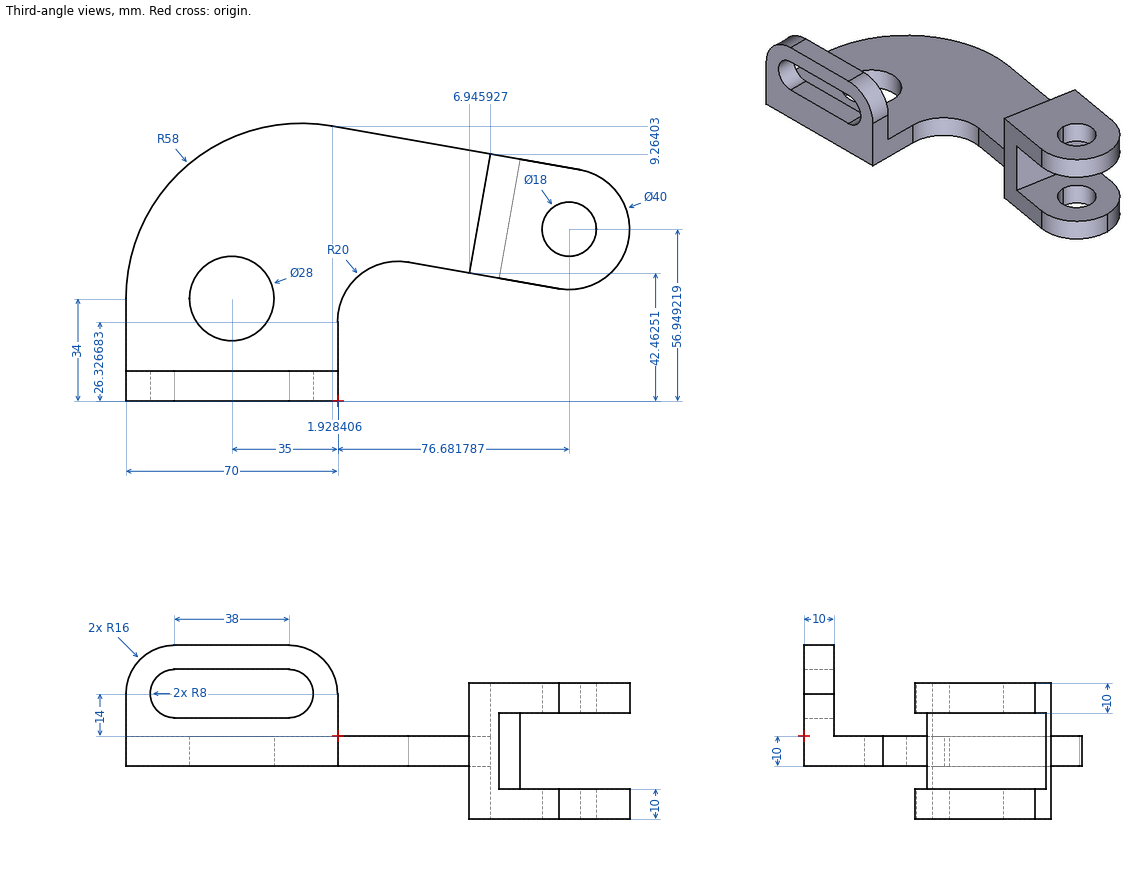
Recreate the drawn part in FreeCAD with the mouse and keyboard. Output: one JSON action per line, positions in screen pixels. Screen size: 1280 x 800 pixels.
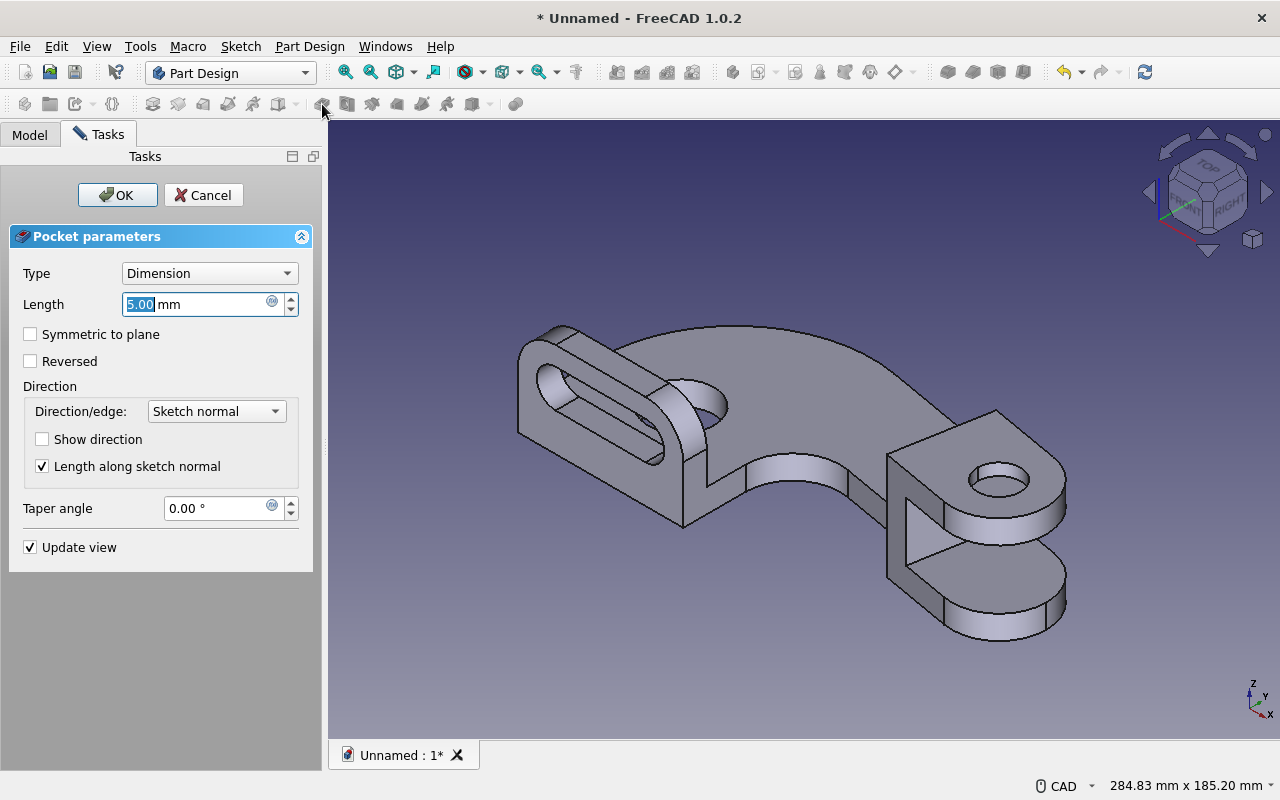
{"action": "left_click", "coordinate": [210, 274]}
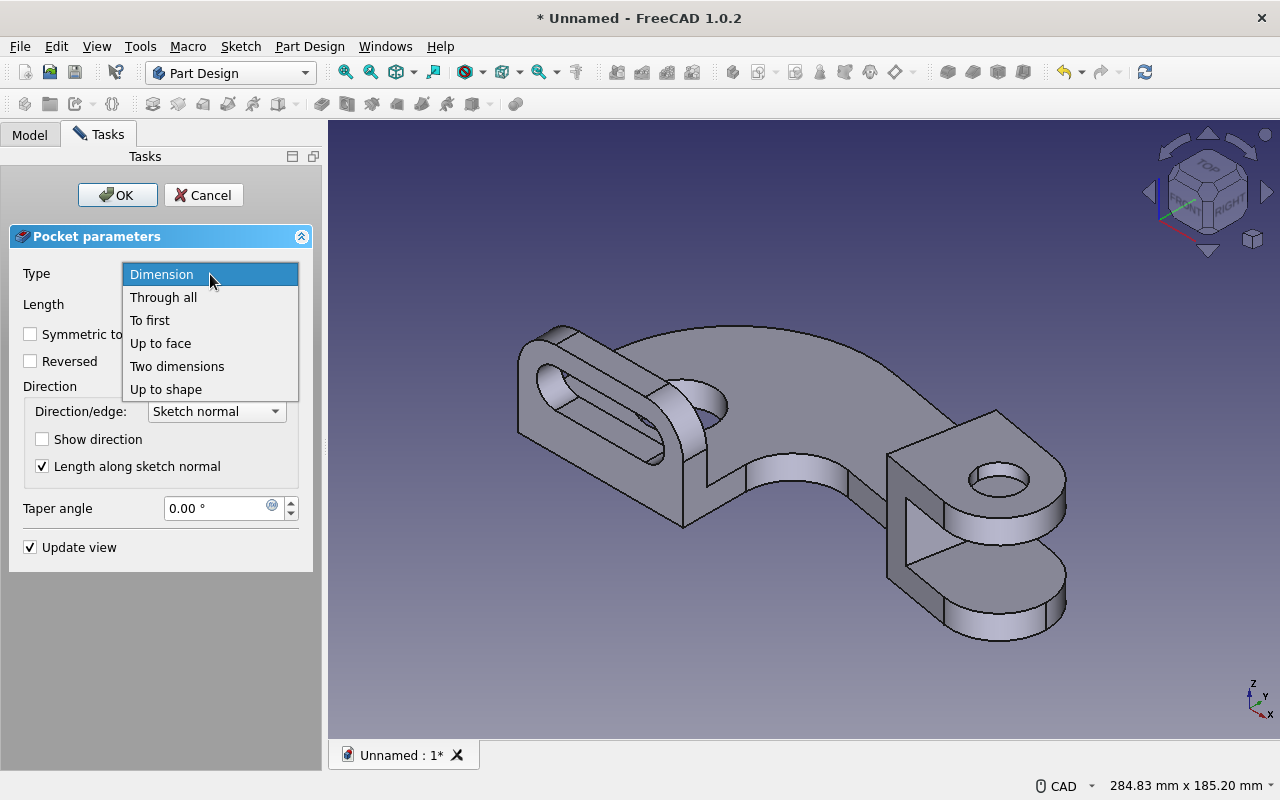
{"action": "left_click", "coordinate": [208, 298]}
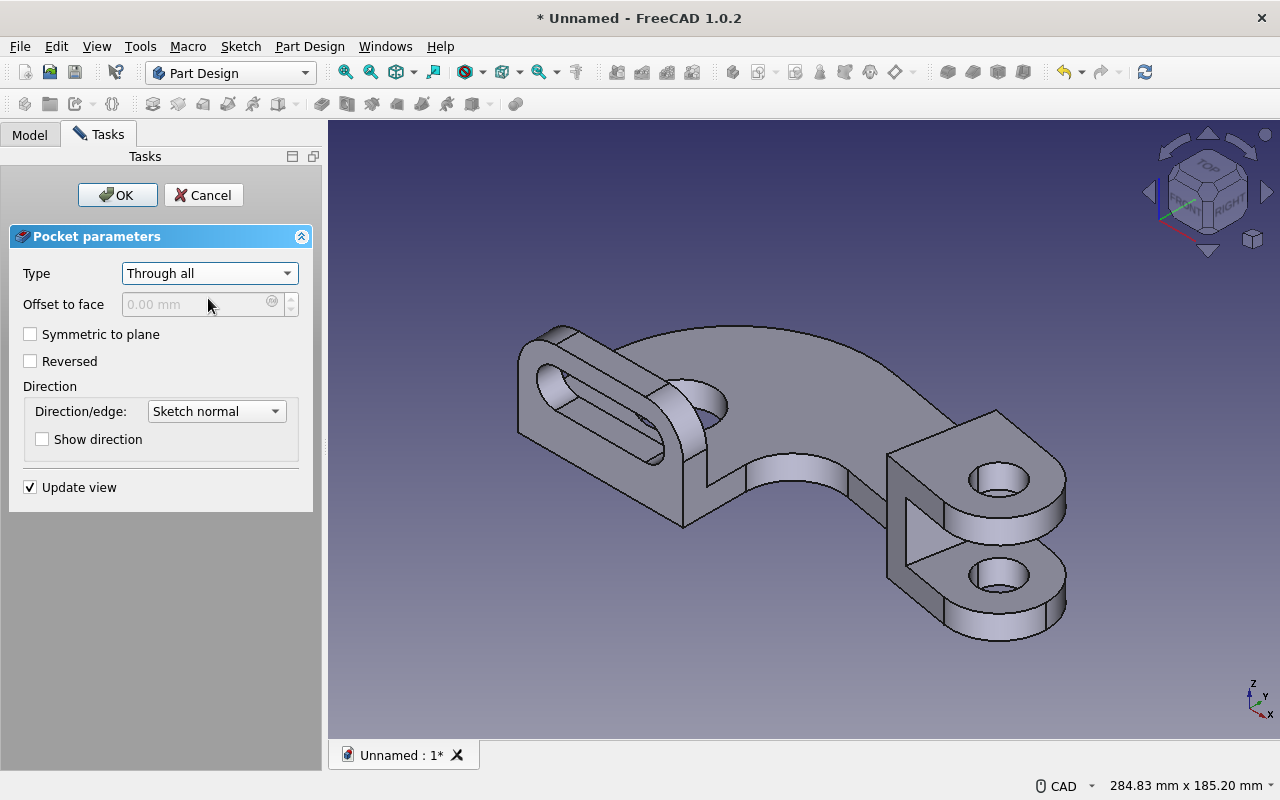
{"action": "left_click", "coordinate": [118, 195]}